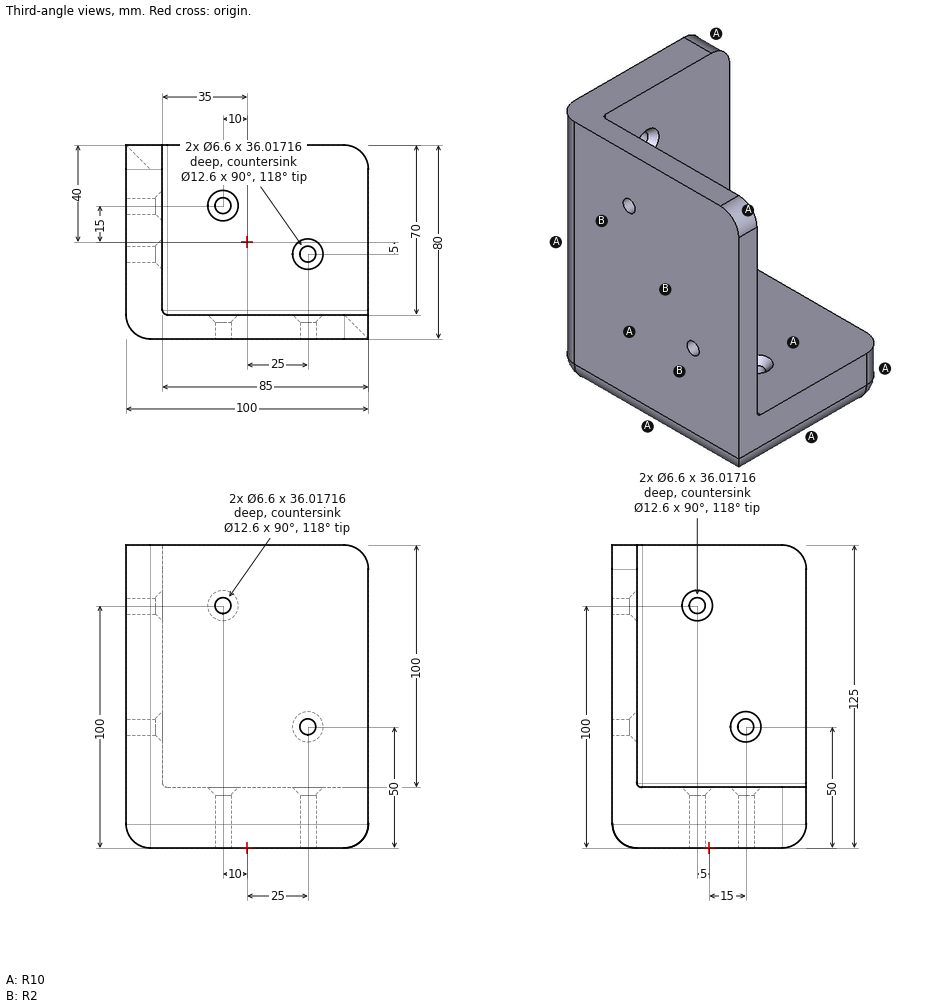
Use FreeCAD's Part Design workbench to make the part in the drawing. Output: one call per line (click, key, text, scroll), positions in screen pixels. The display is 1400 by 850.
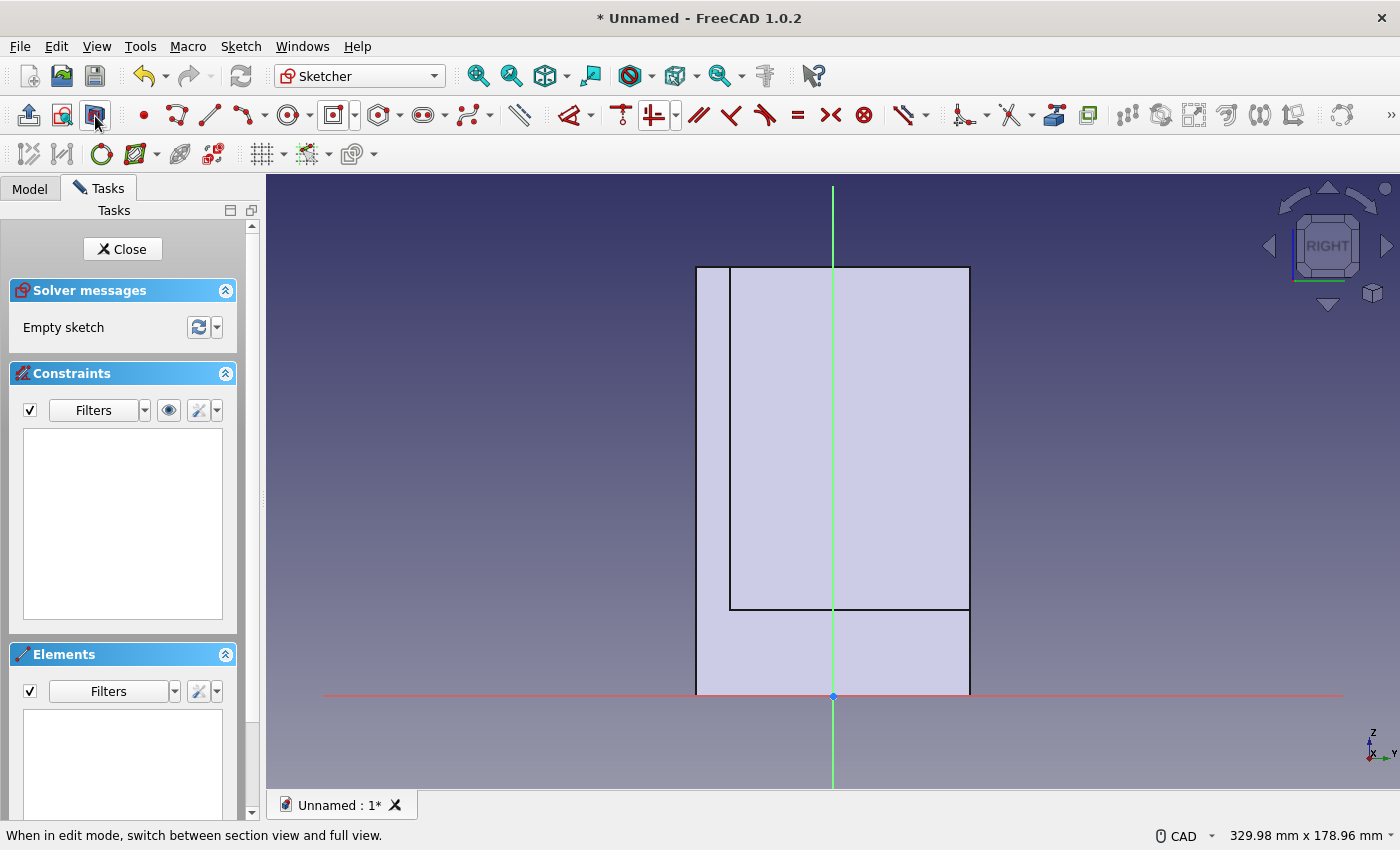
key(g)
key(c)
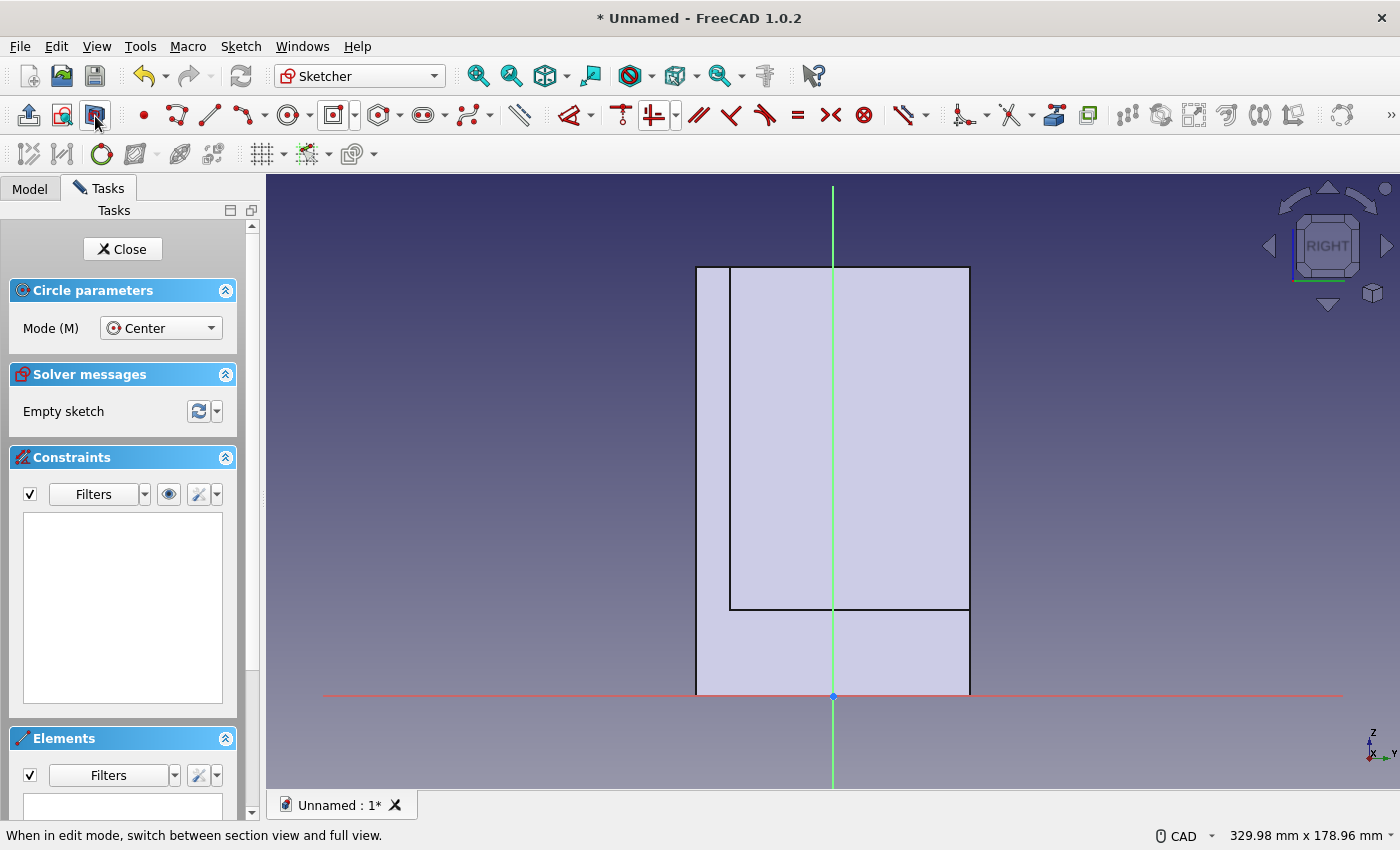
scroll(816, 353, up, 4)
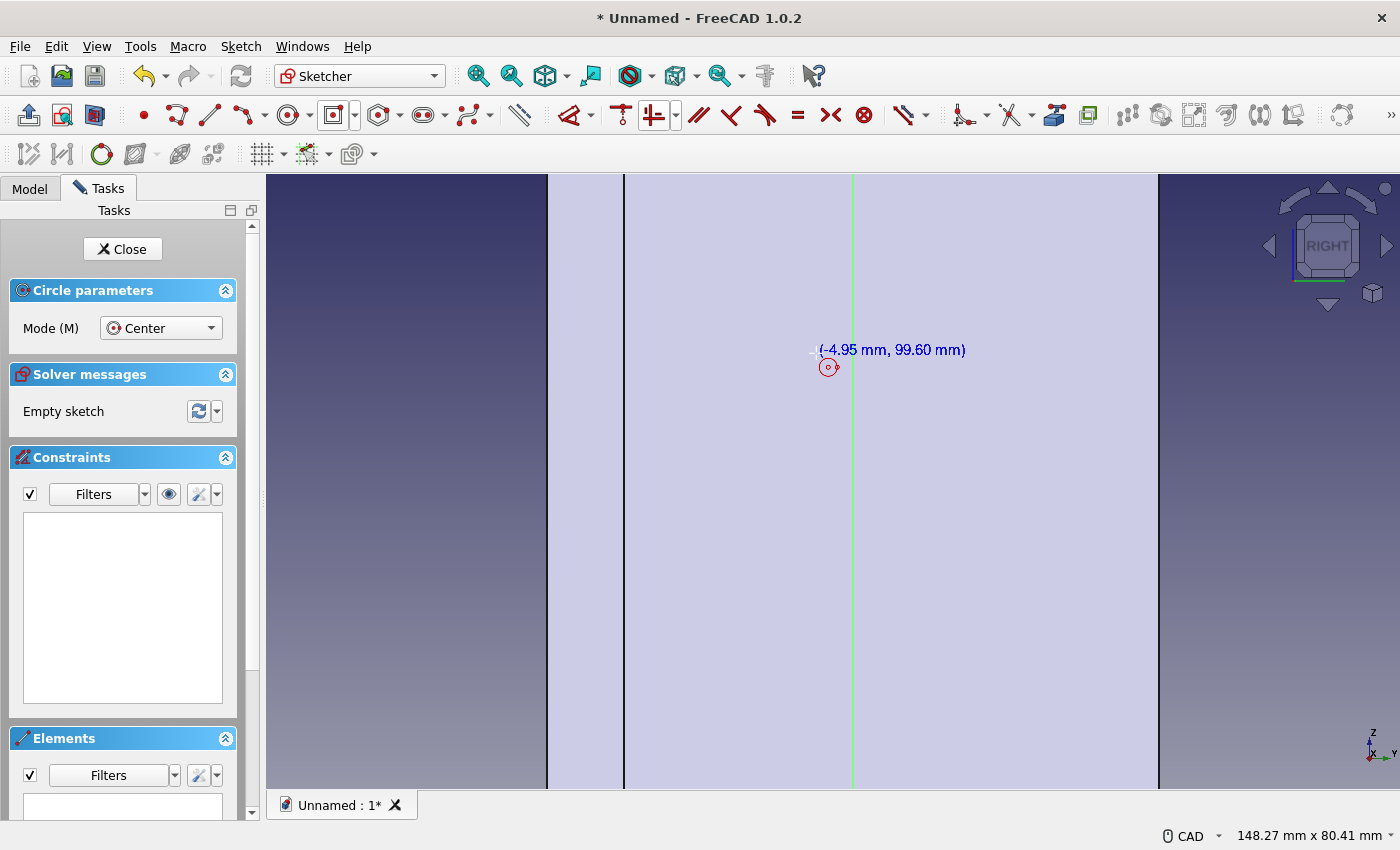
click(815, 352)
move(833, 334)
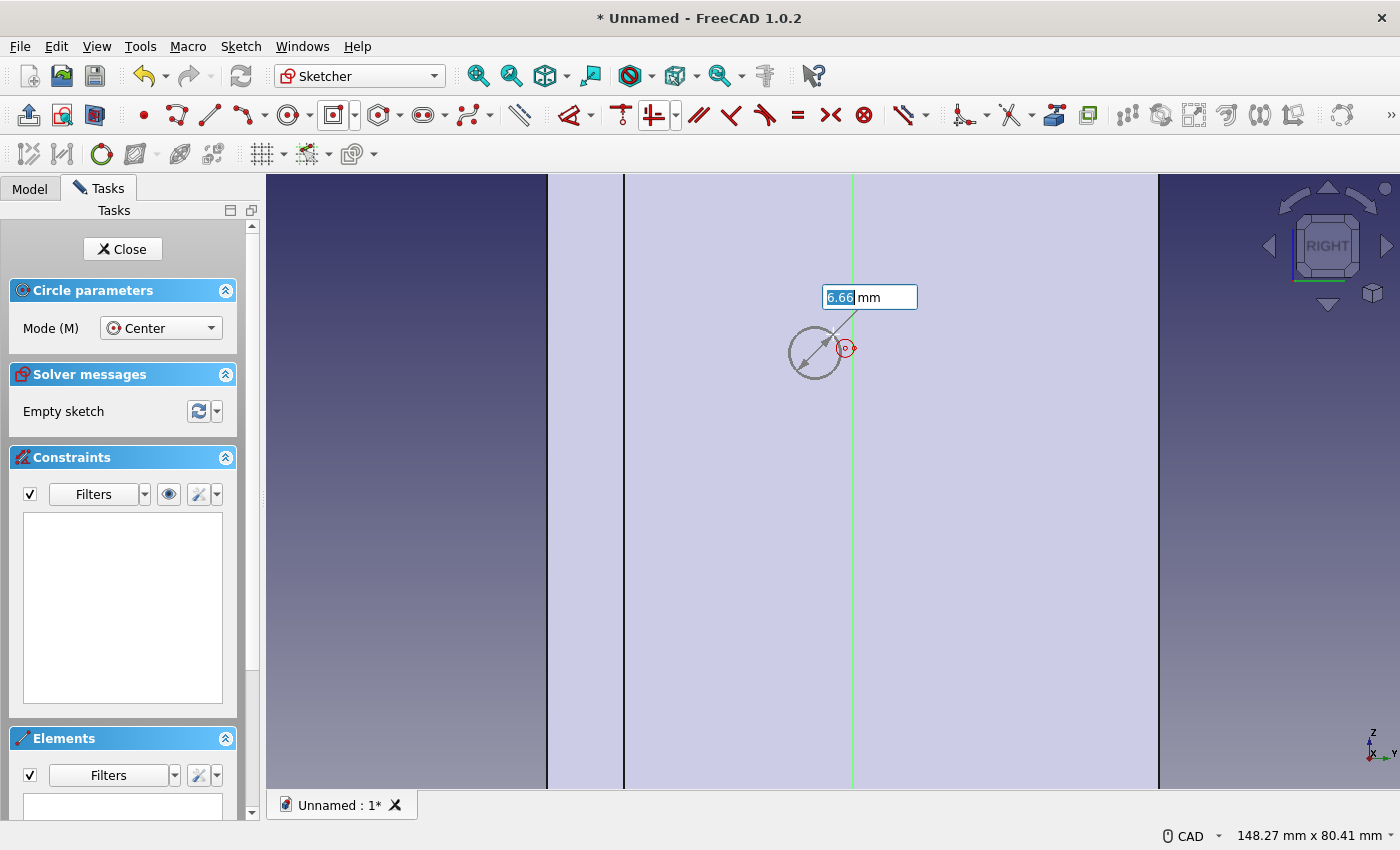
text(6.6)
key(Return)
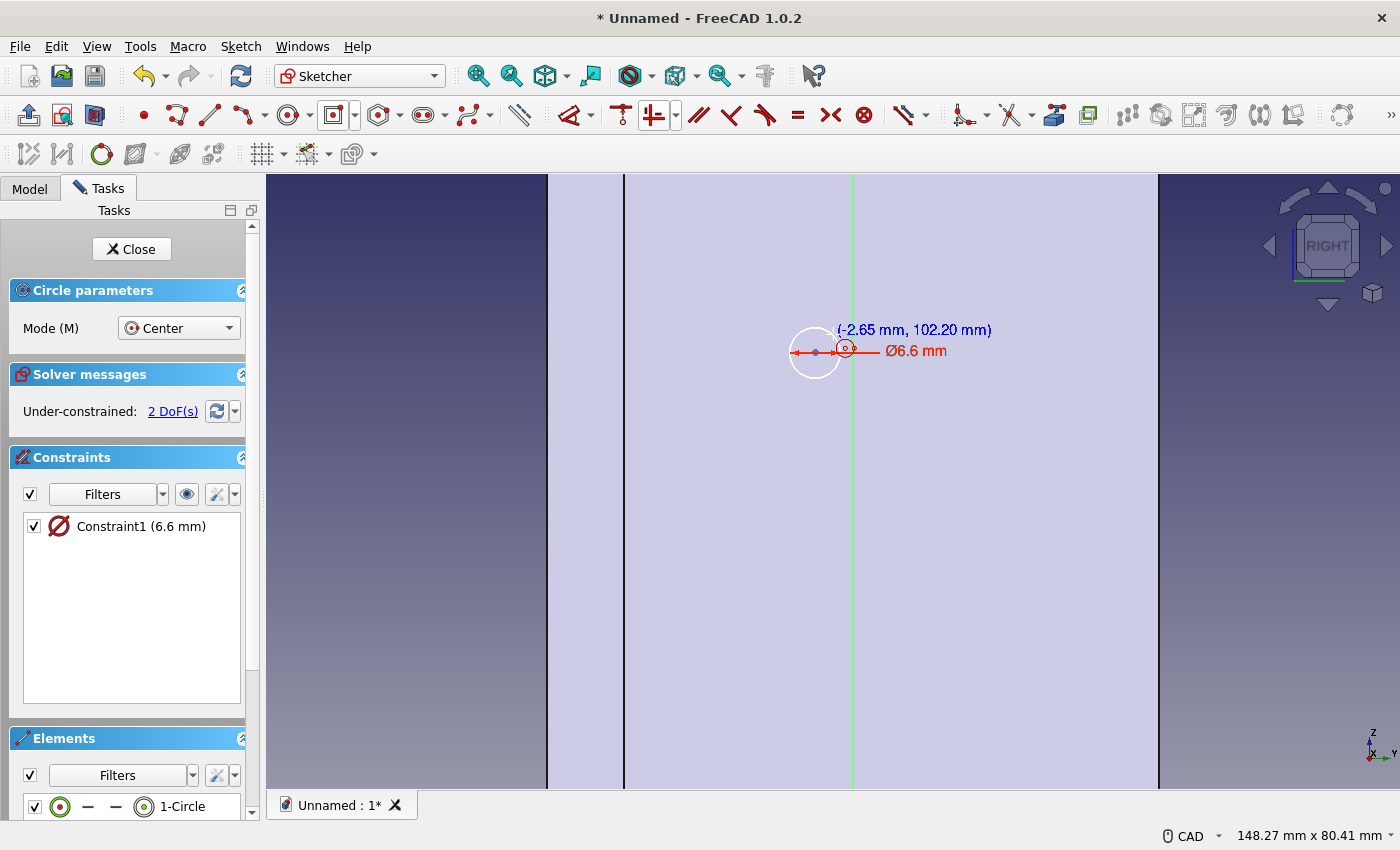
click(968, 734)
move(986, 716)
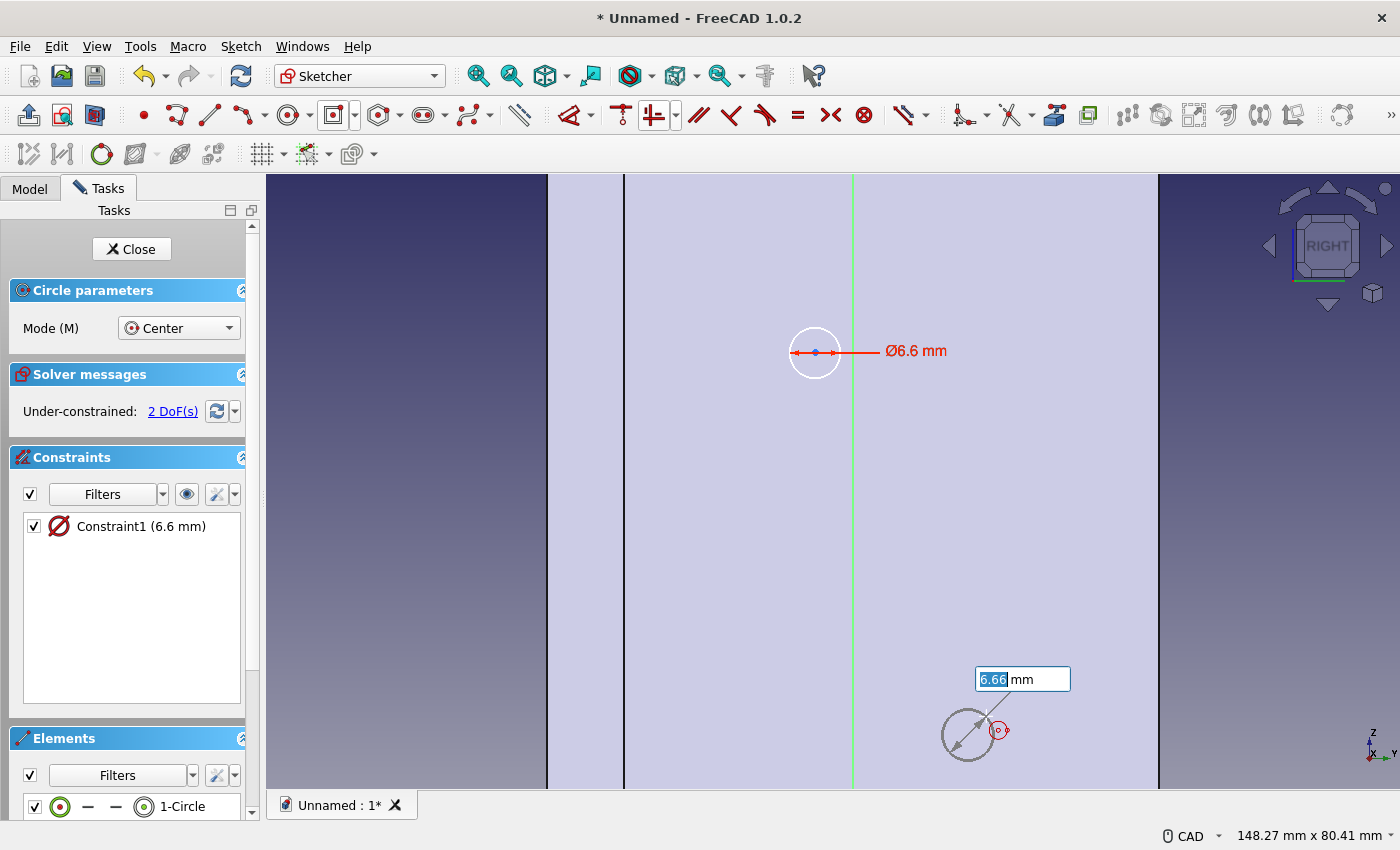
text(6.6)
key(Return)
key(Escape)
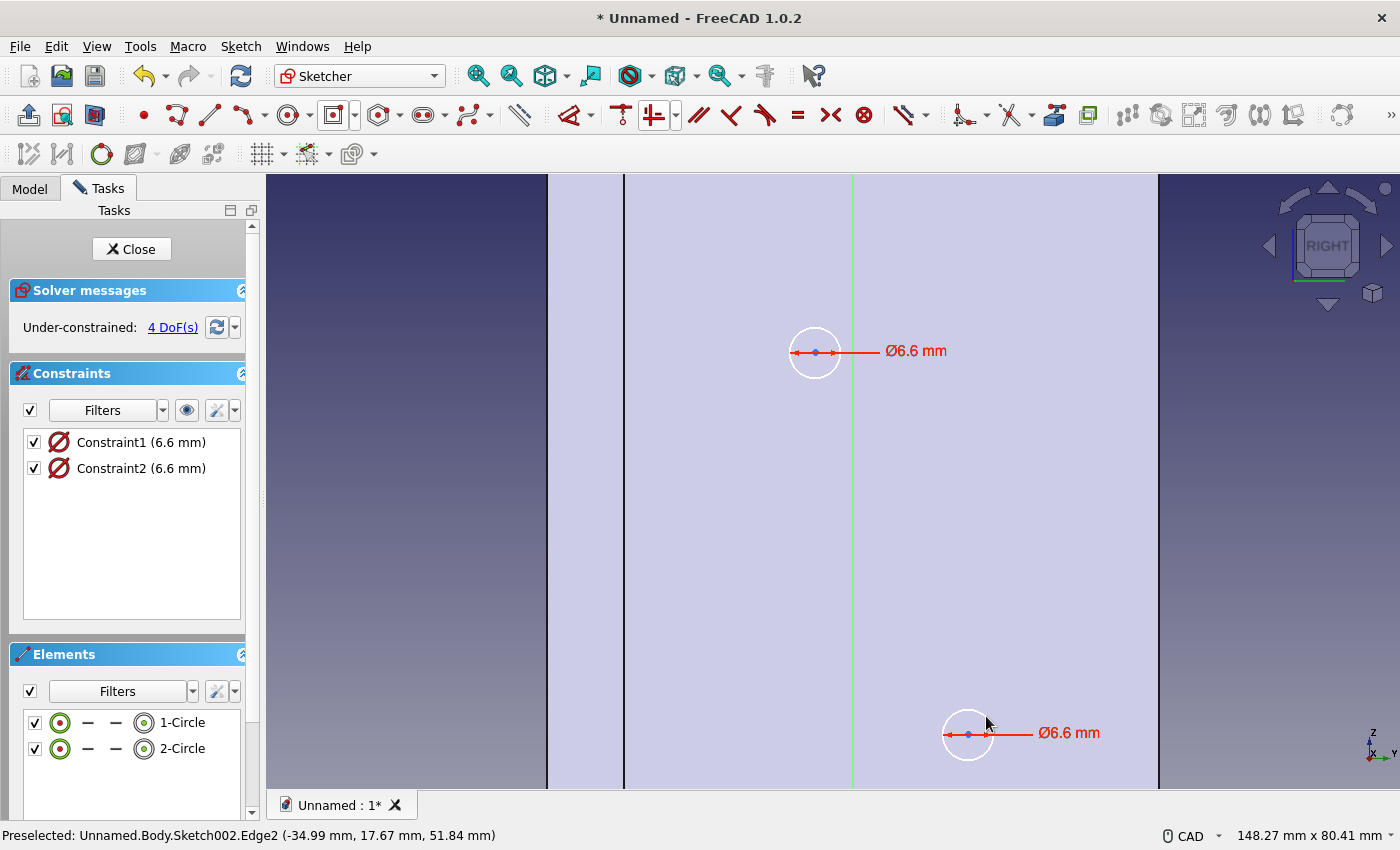
click(568, 116)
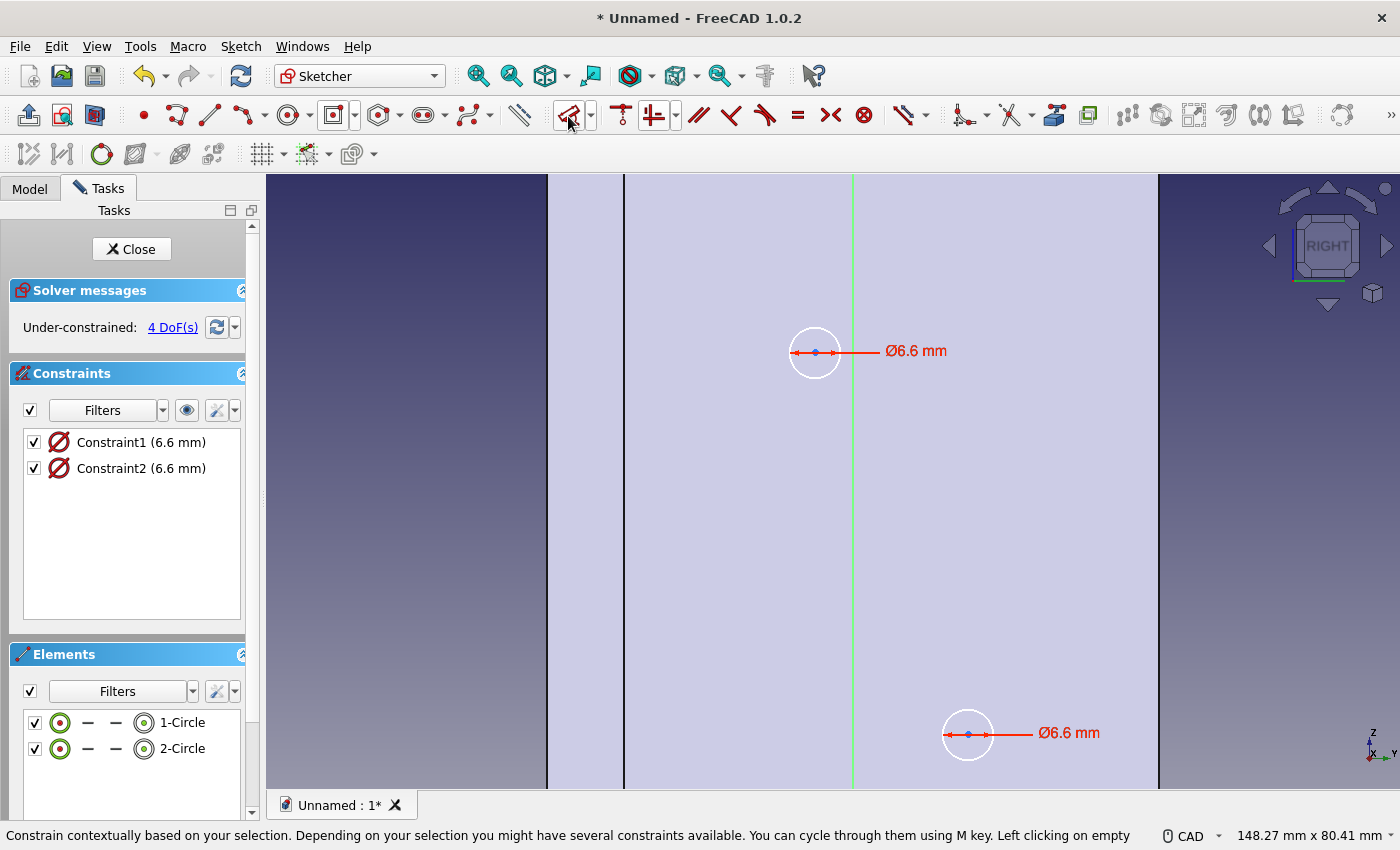
click(815, 353)
click(834, 319)